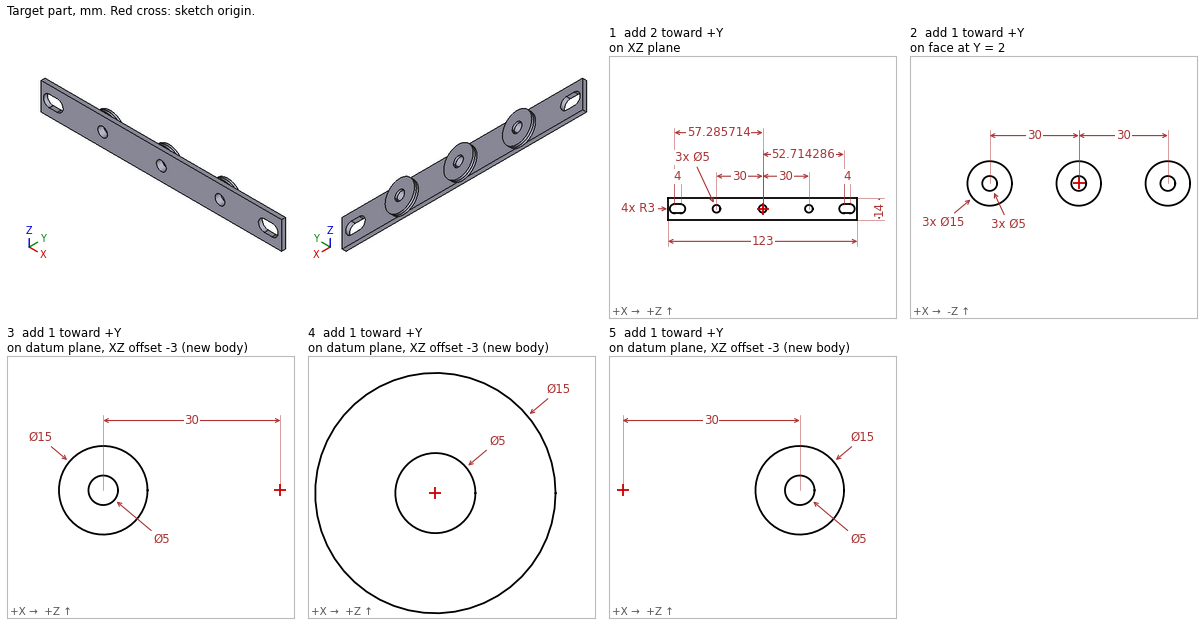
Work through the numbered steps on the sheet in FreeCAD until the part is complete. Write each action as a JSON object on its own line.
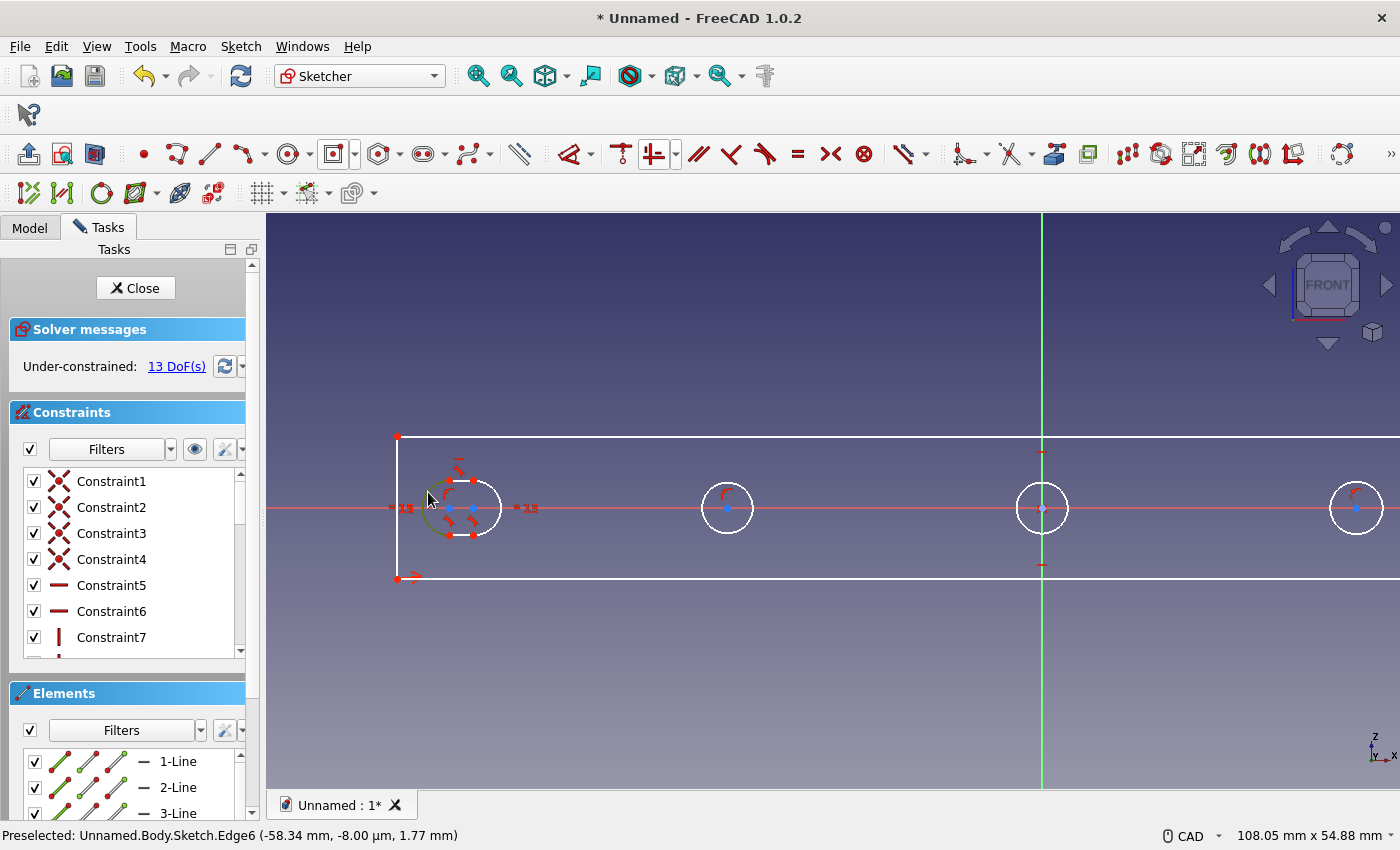
{"action": "scroll", "coordinate": [427, 492], "scroll_direction": "down", "scroll_amount": 3}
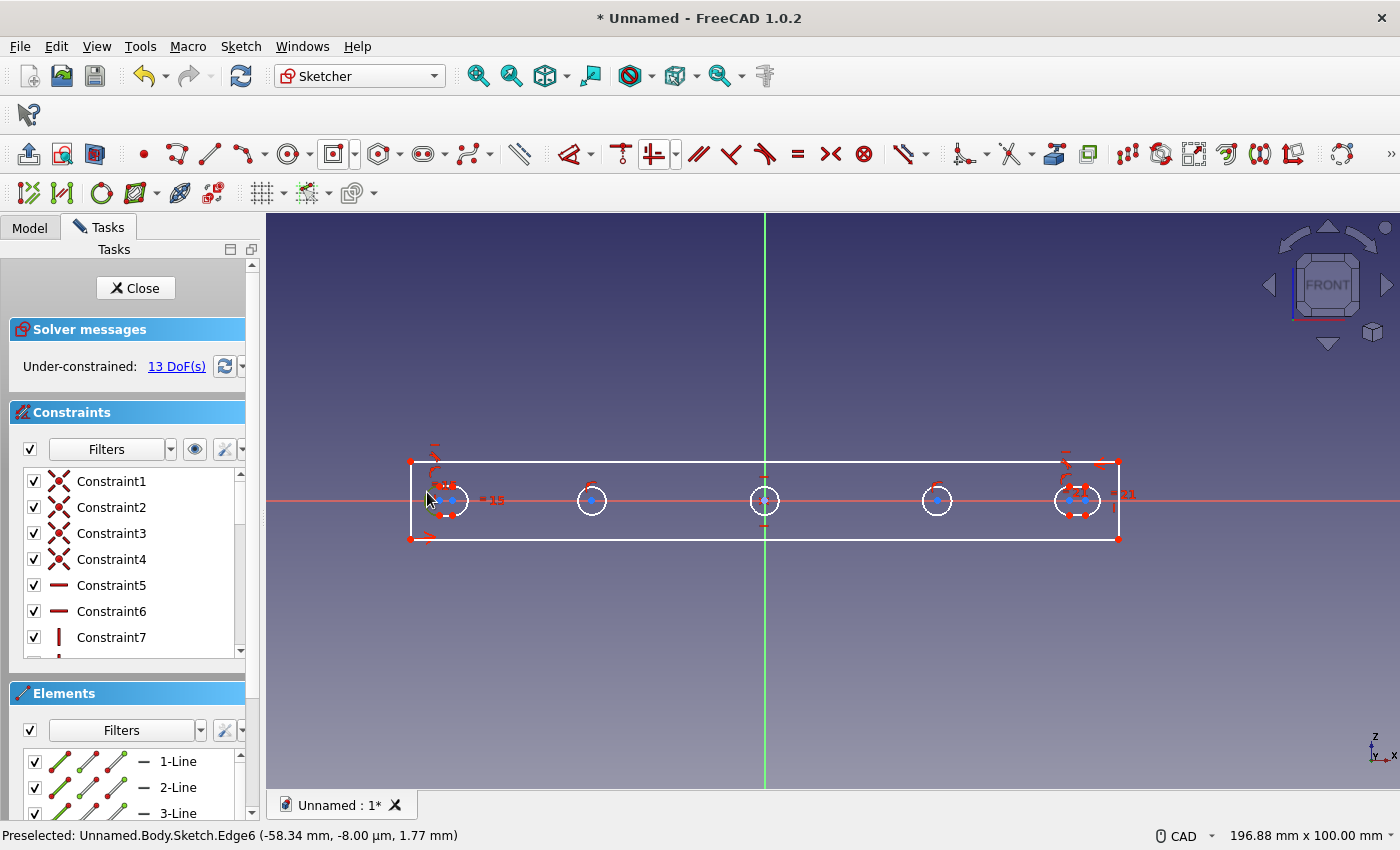
{"action": "scroll", "coordinate": [1058, 493], "scroll_direction": "up", "scroll_amount": 3}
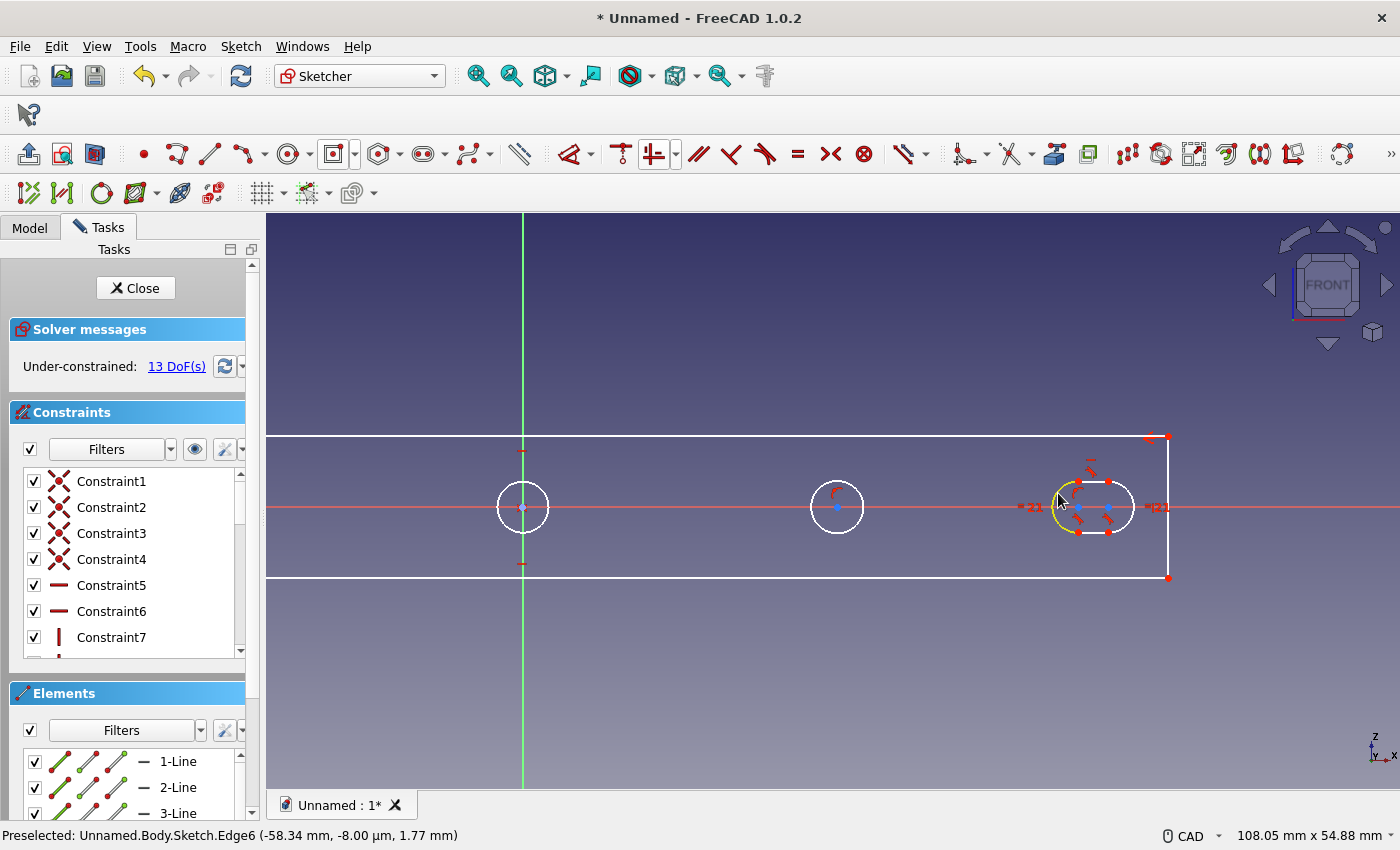
{"action": "left_click", "coordinate": [1057, 492]}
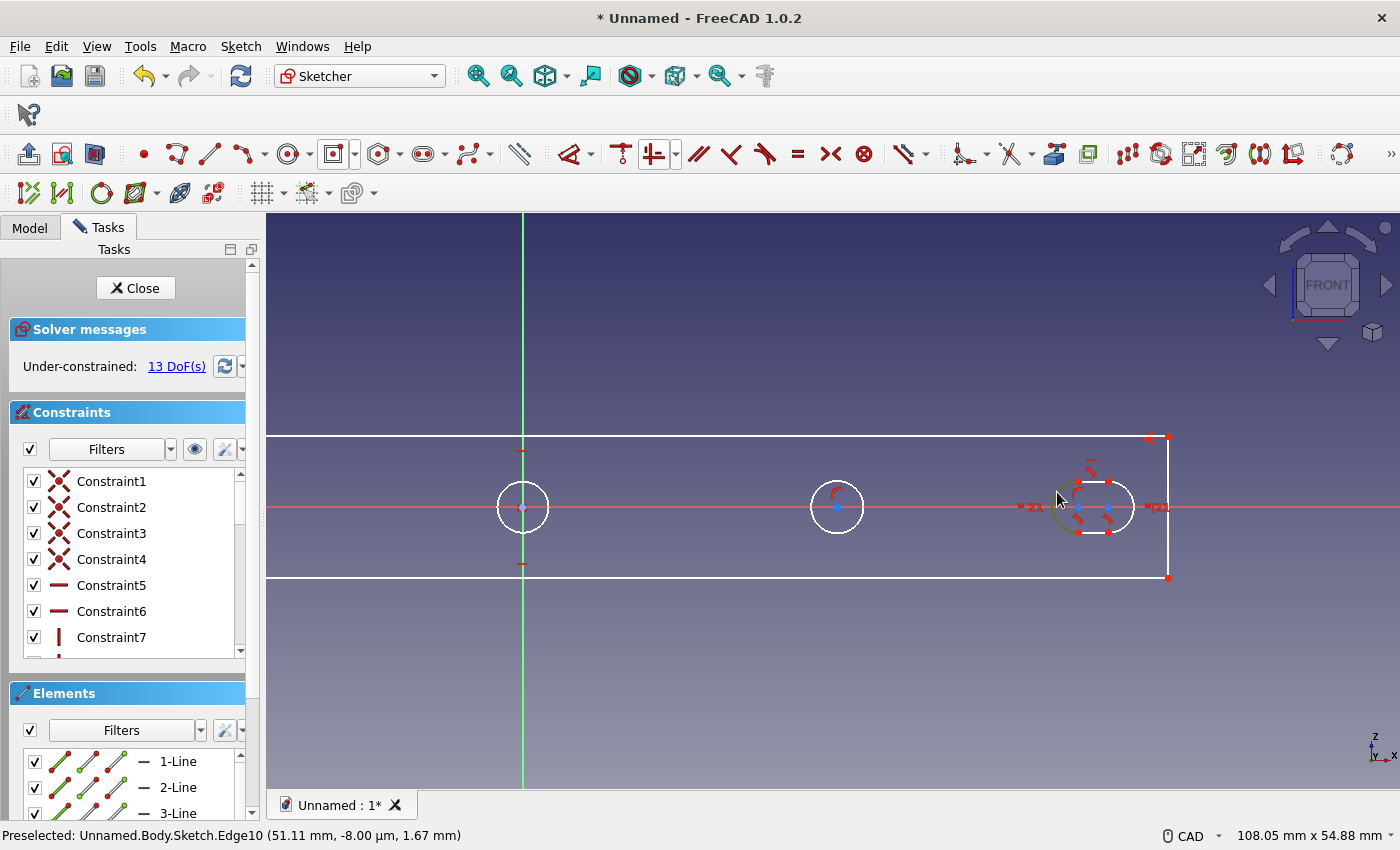
{"action": "left_click", "coordinate": [798, 154]}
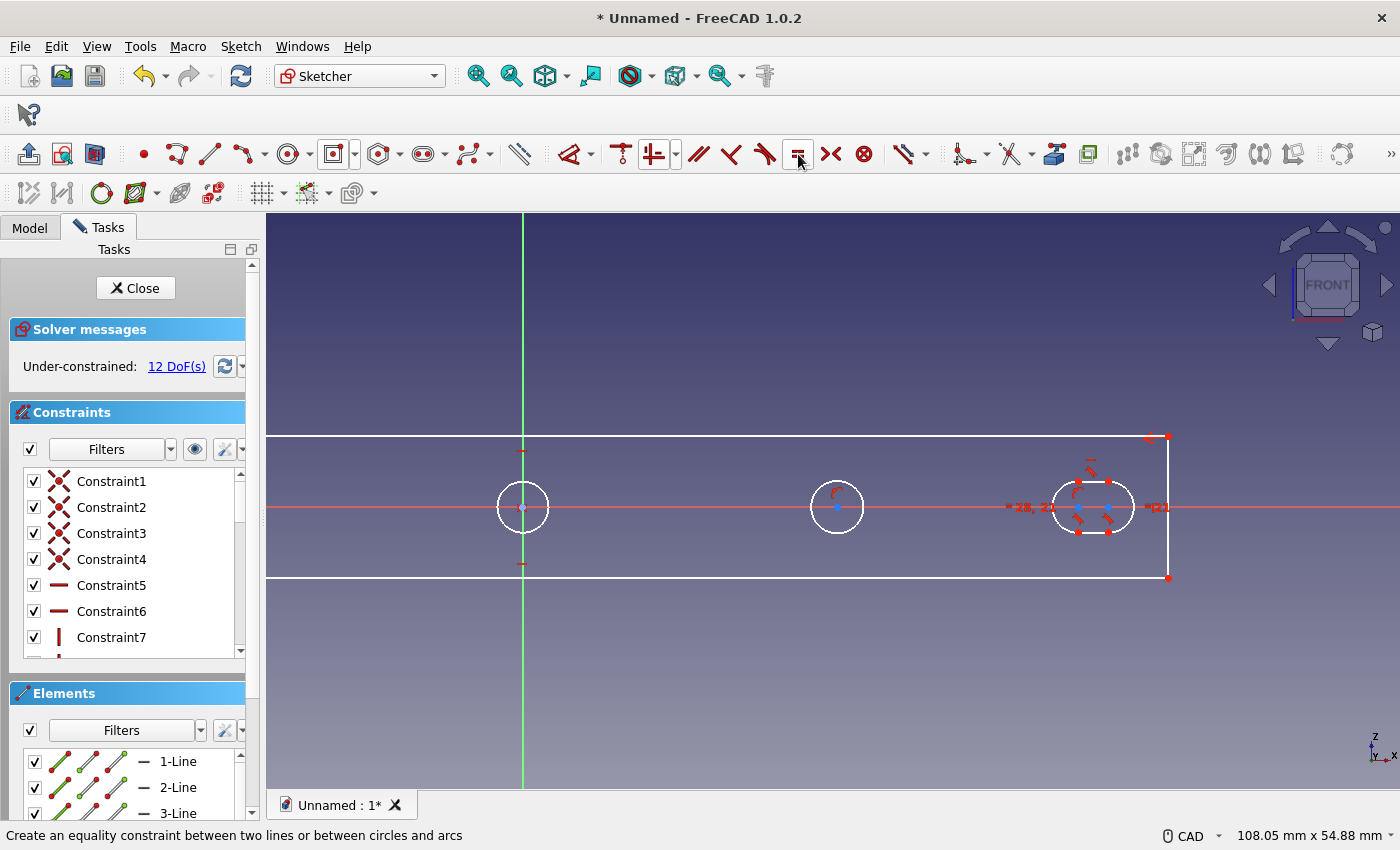
{"action": "scroll", "coordinate": [1058, 493], "scroll_direction": "down", "scroll_amount": 3}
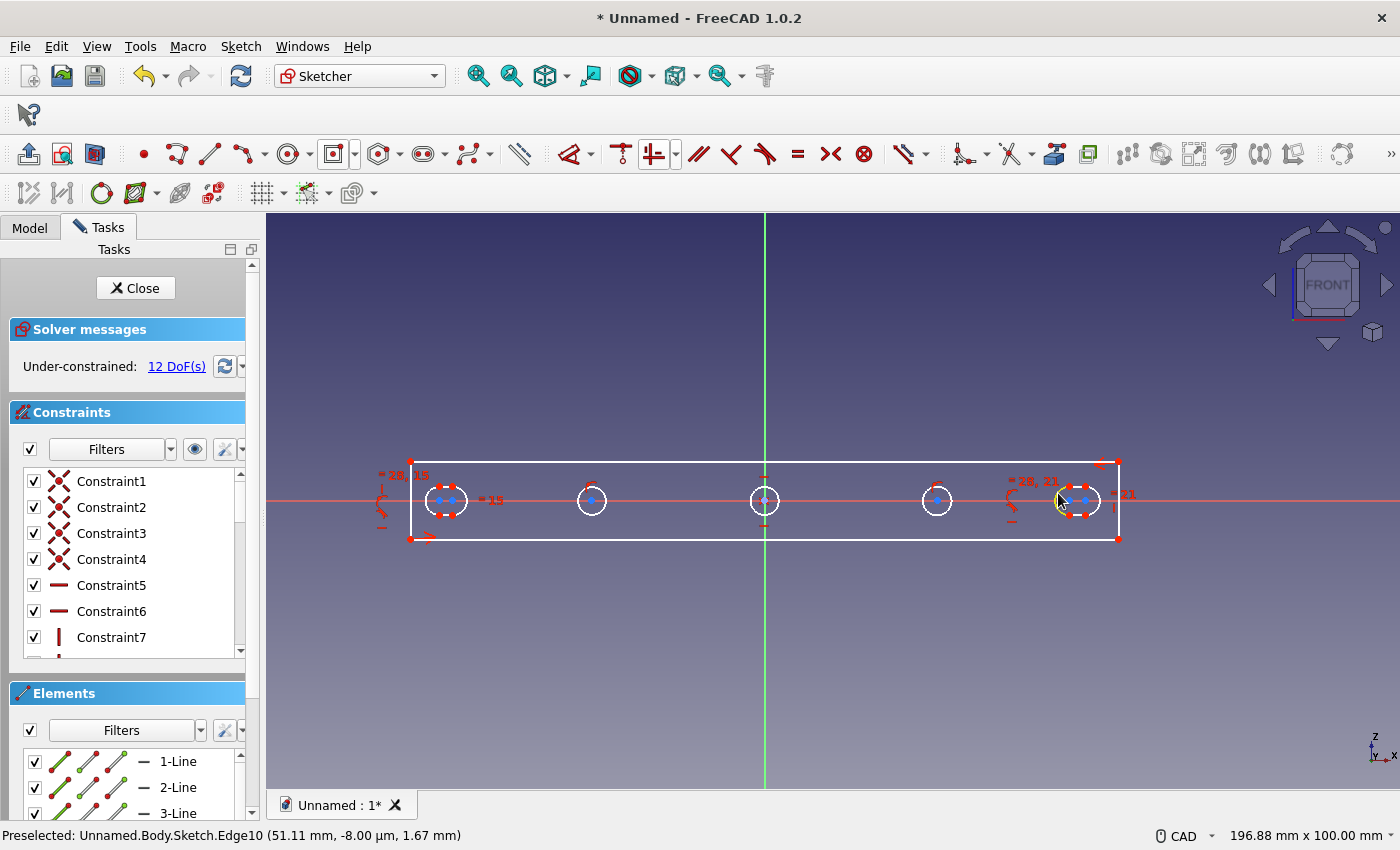
{"action": "scroll", "coordinate": [602, 491], "scroll_direction": "up", "scroll_amount": 2}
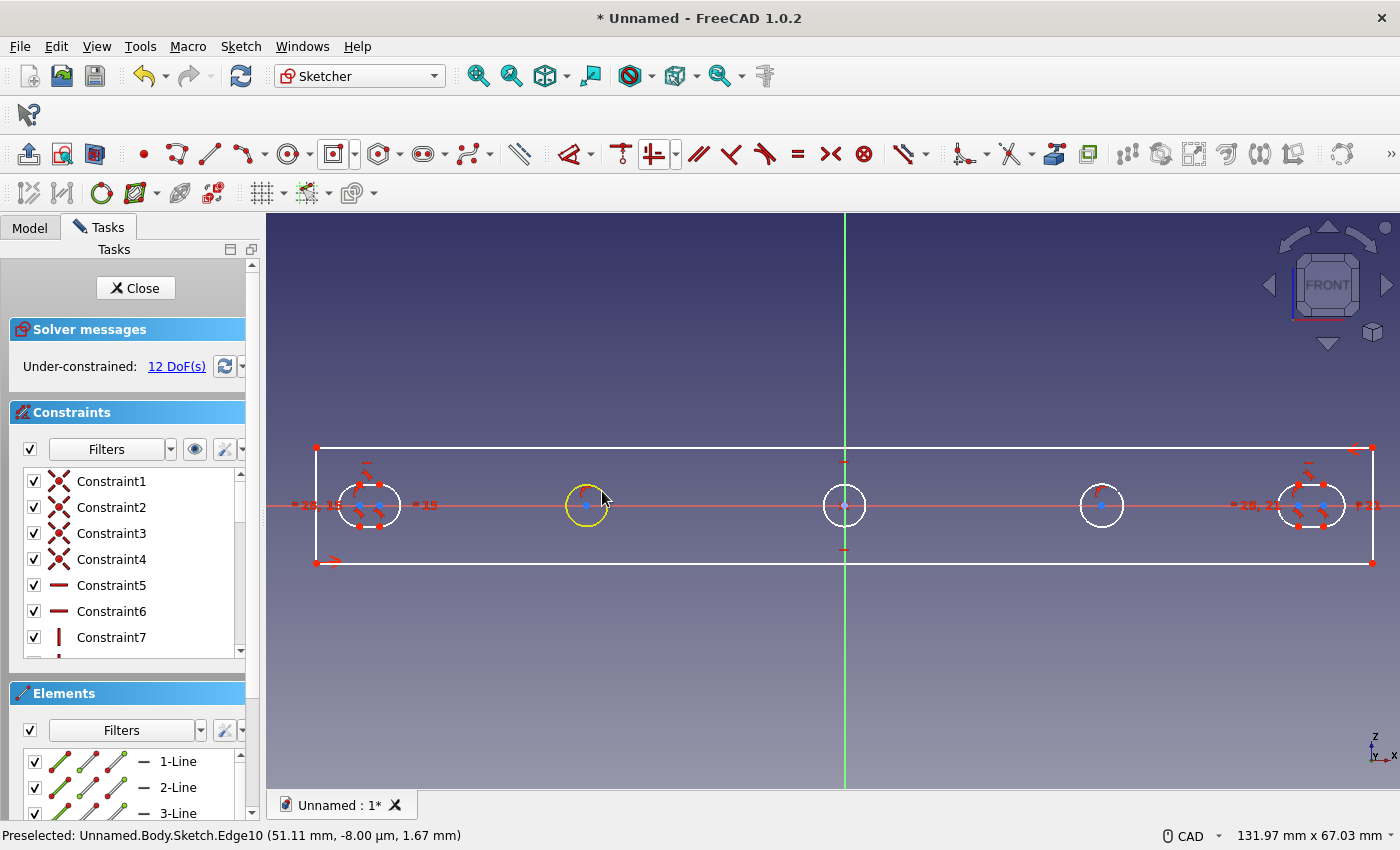
{"action": "left_click", "coordinate": [601, 491]}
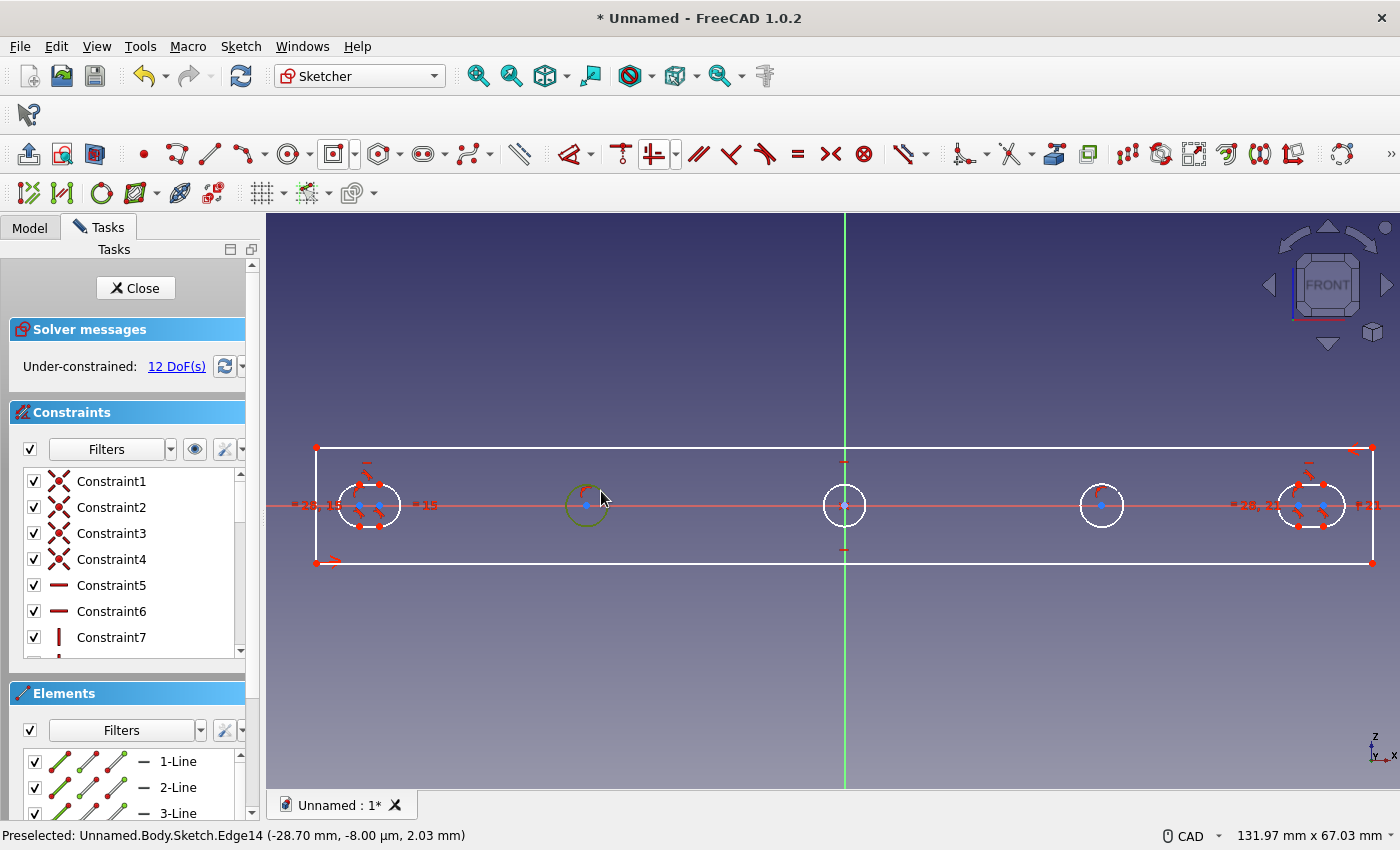
{"action": "left_click", "coordinate": [859, 491]}